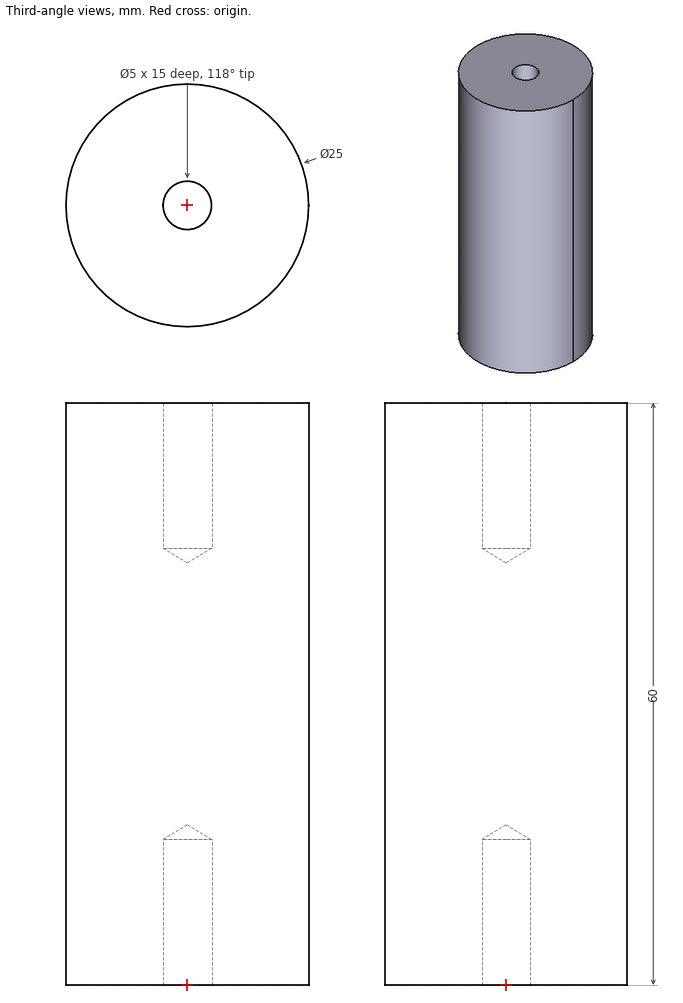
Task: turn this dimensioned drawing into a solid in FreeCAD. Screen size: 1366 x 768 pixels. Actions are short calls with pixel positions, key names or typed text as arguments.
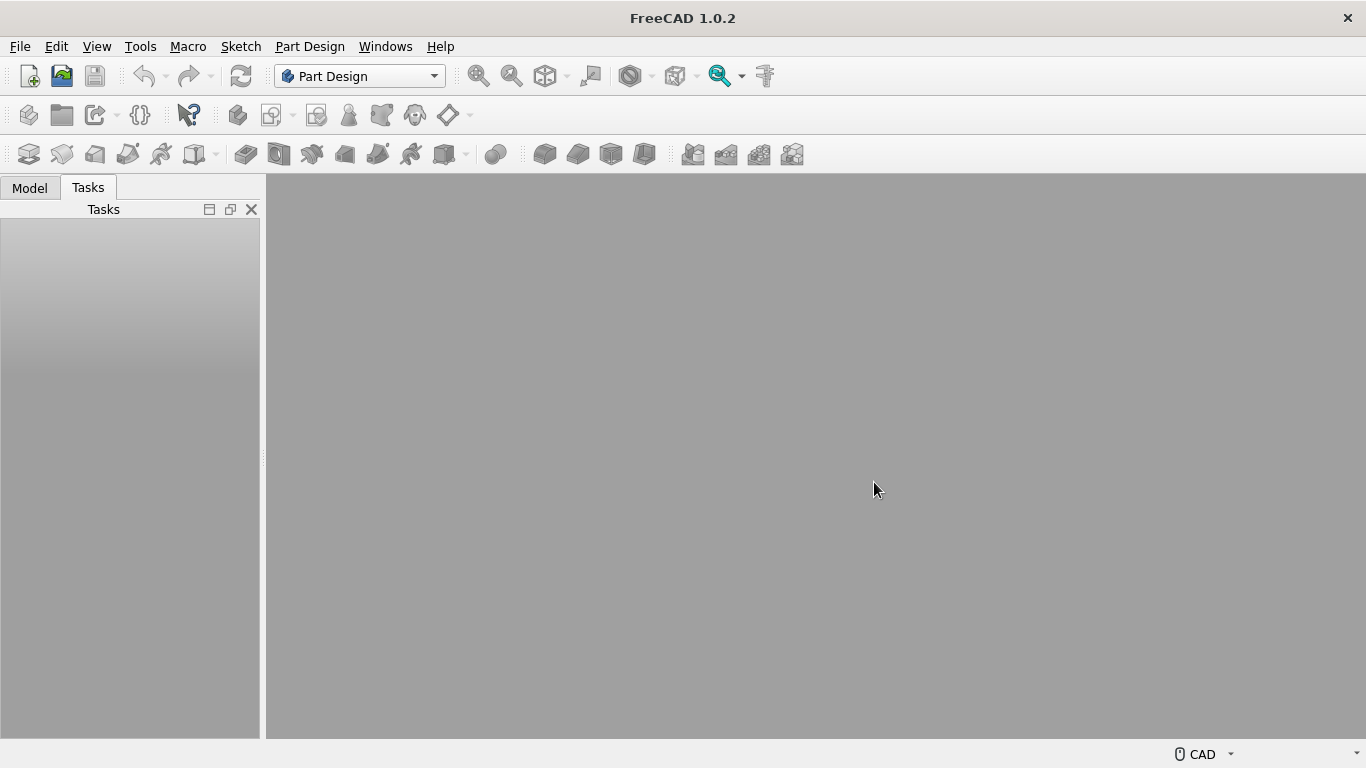
click(29, 76)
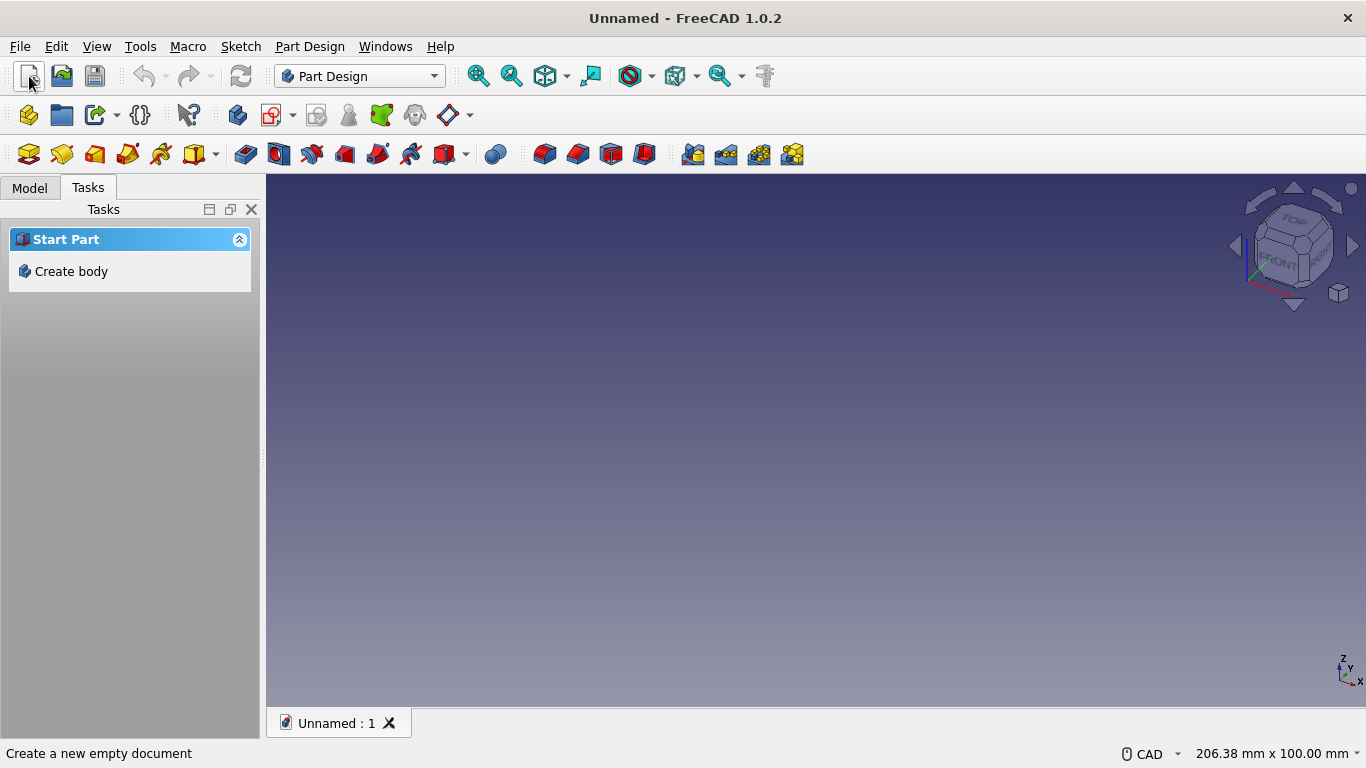
click(270, 116)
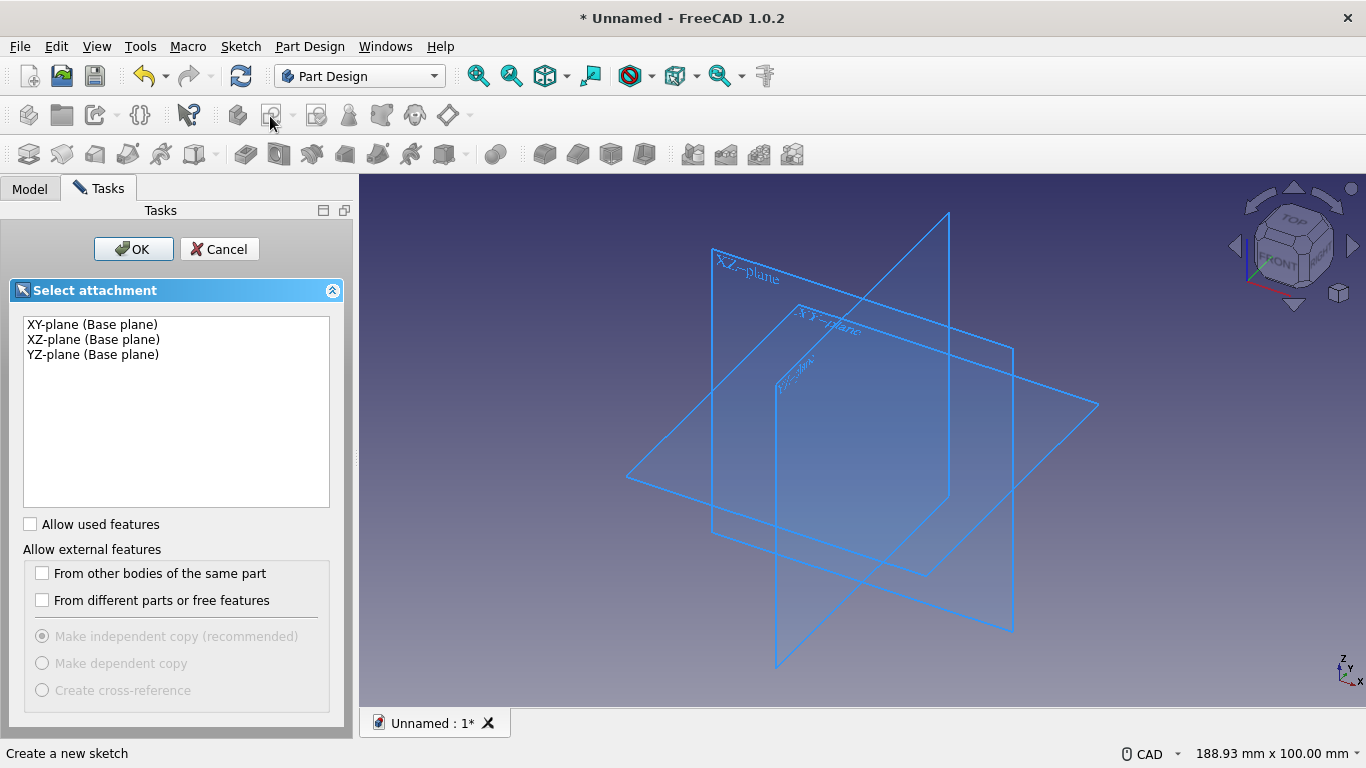
click(84, 324)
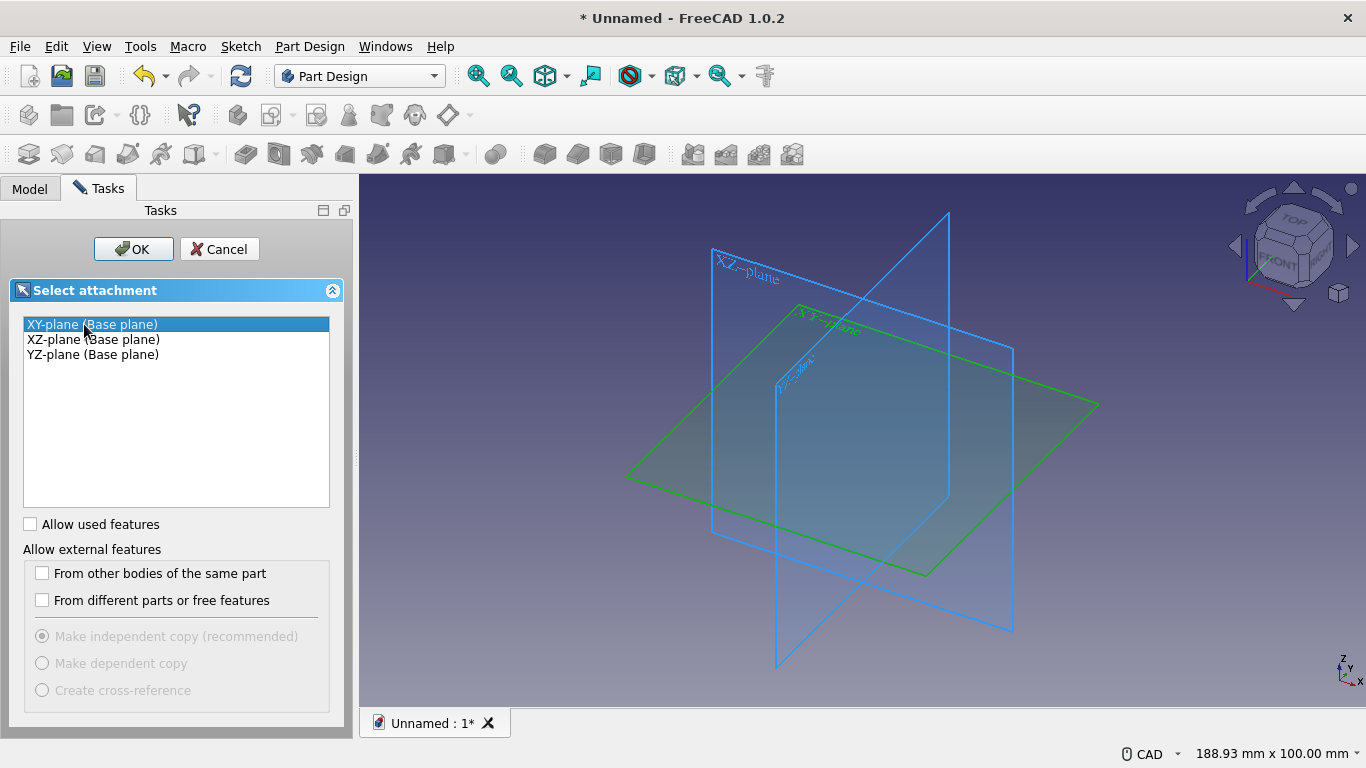
click(134, 249)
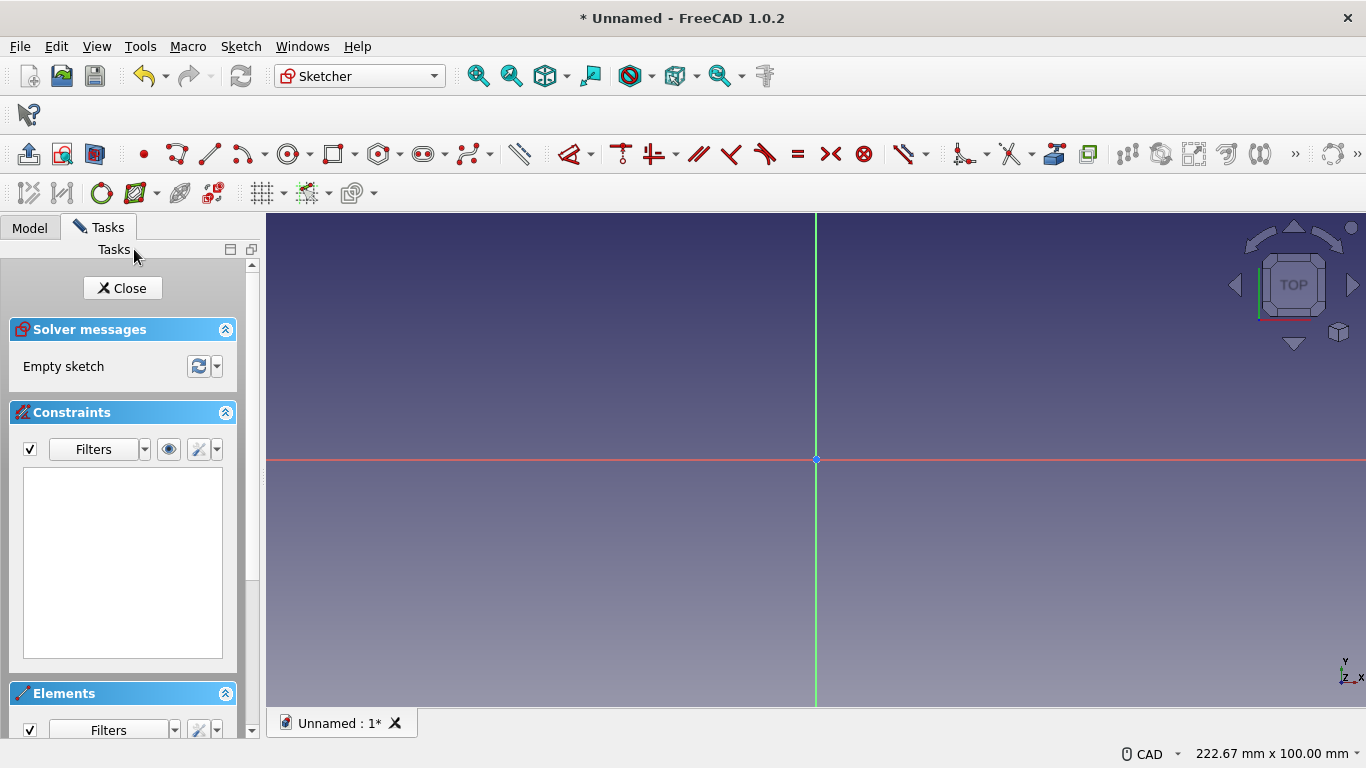
scroll(856, 460, up, 5)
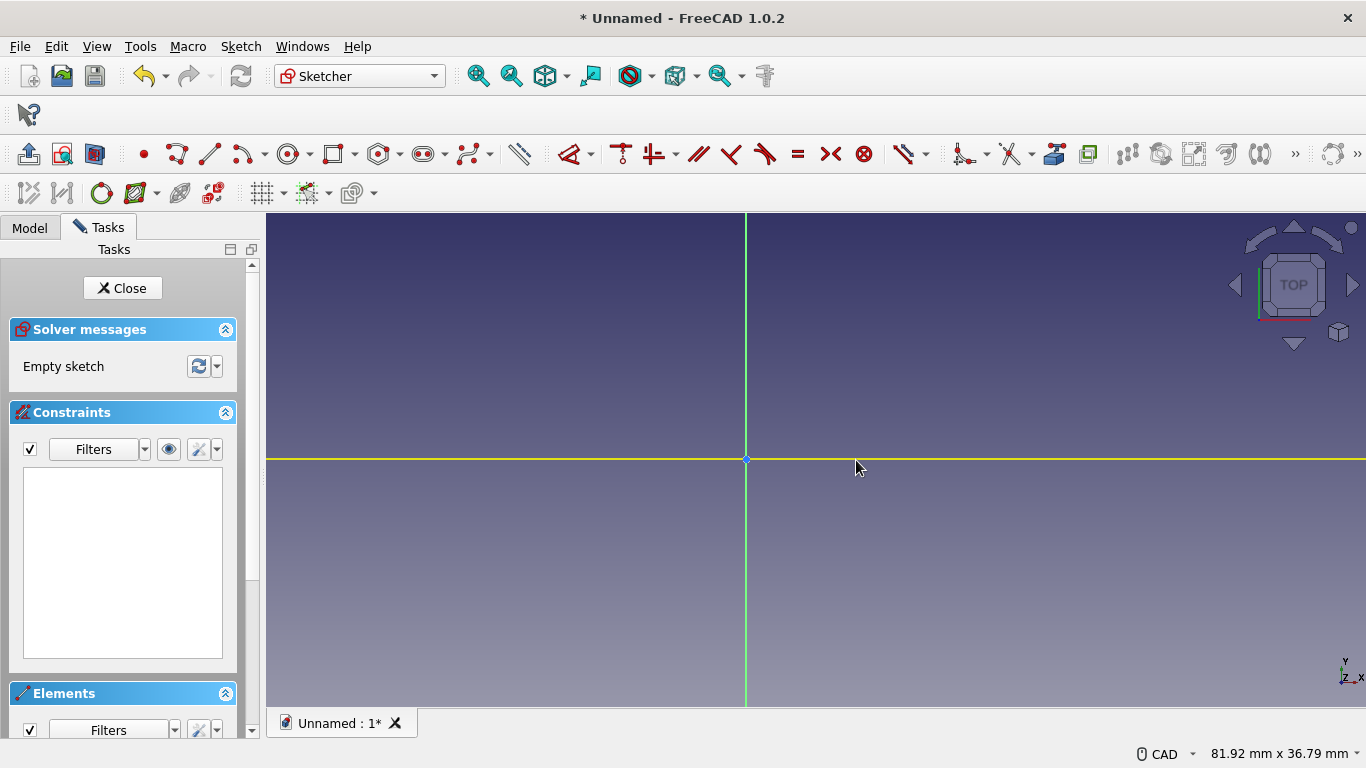
click(288, 154)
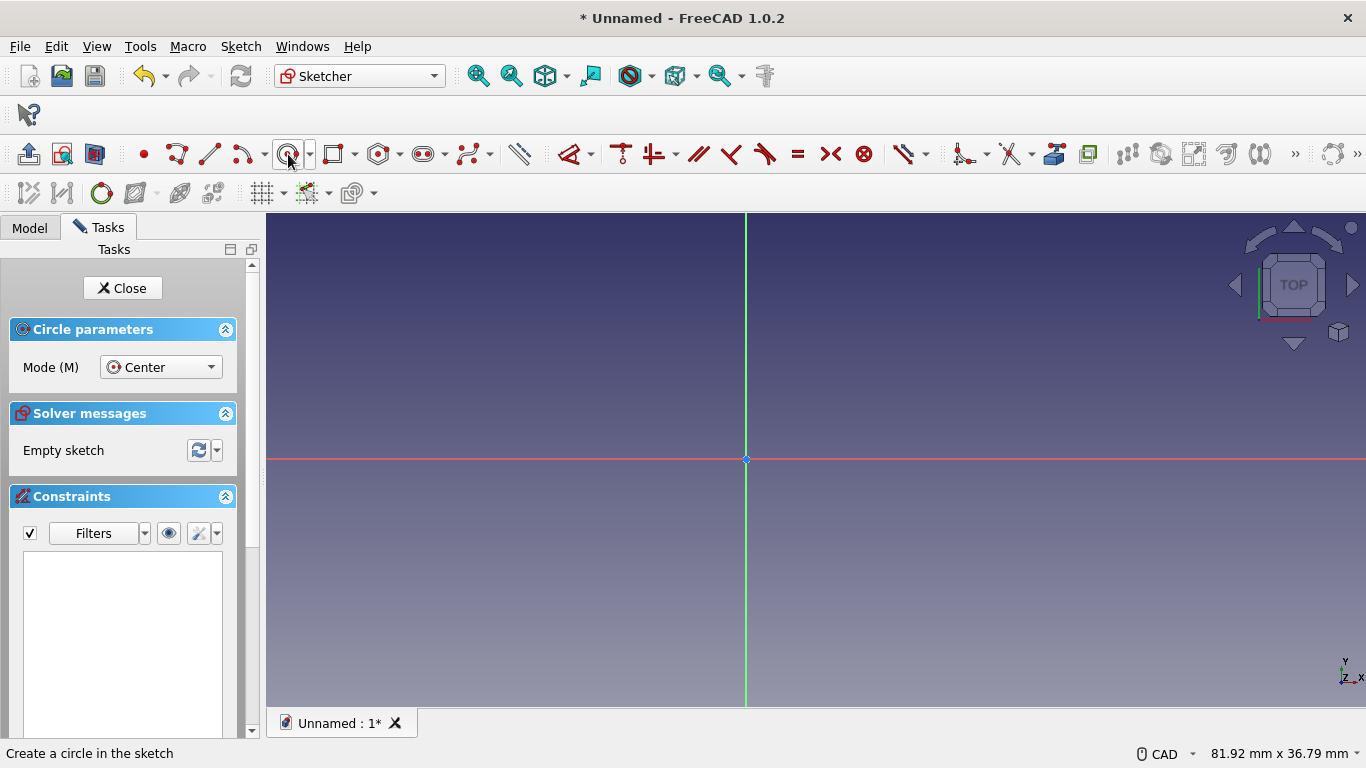
click(746, 459)
click(865, 340)
key(Escape)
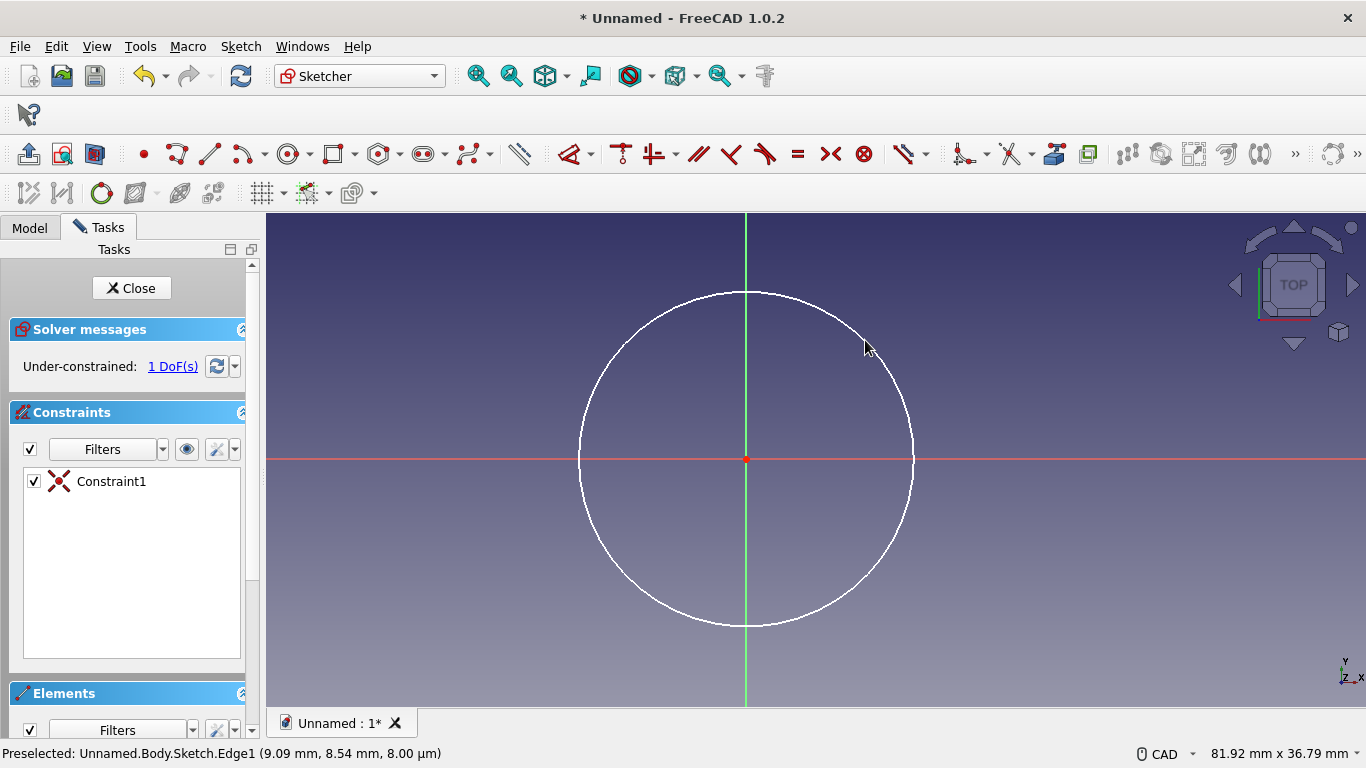
click(568, 154)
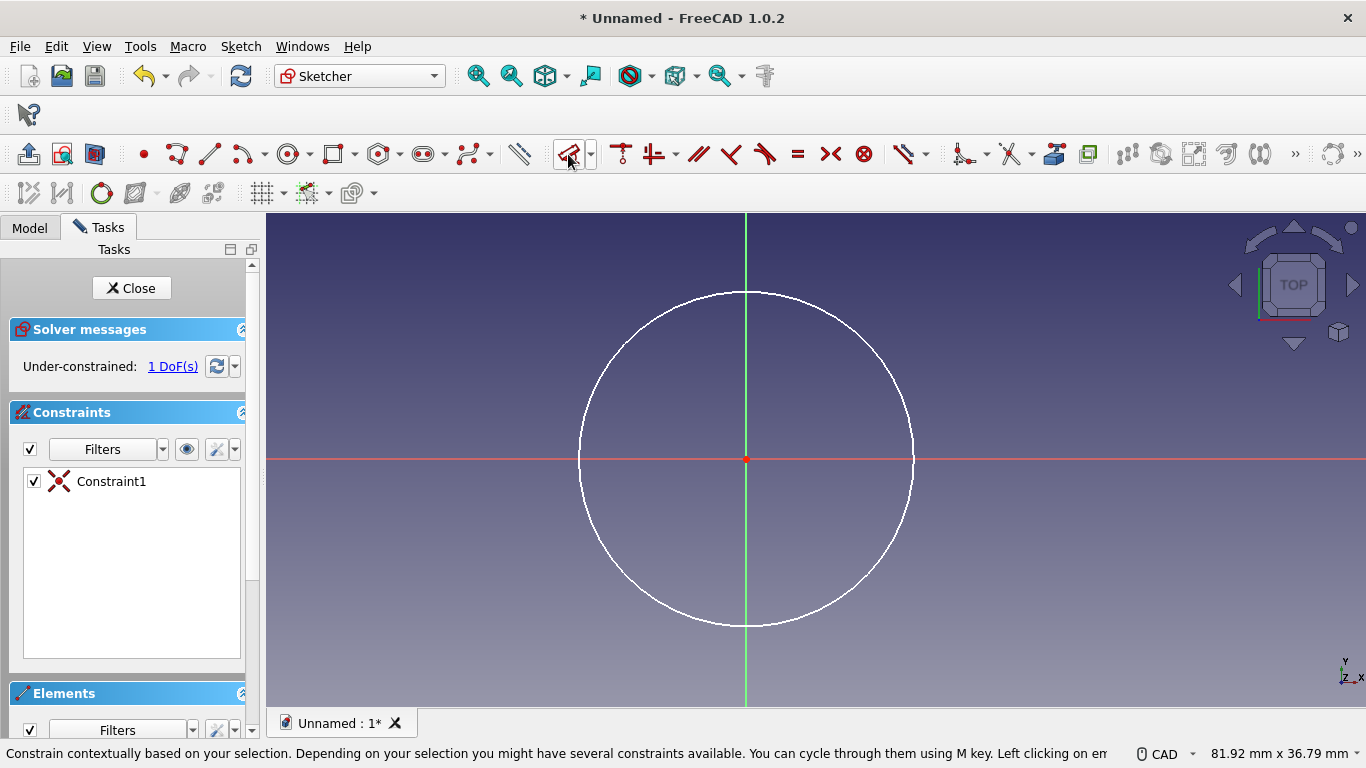
click(864, 340)
click(886, 317)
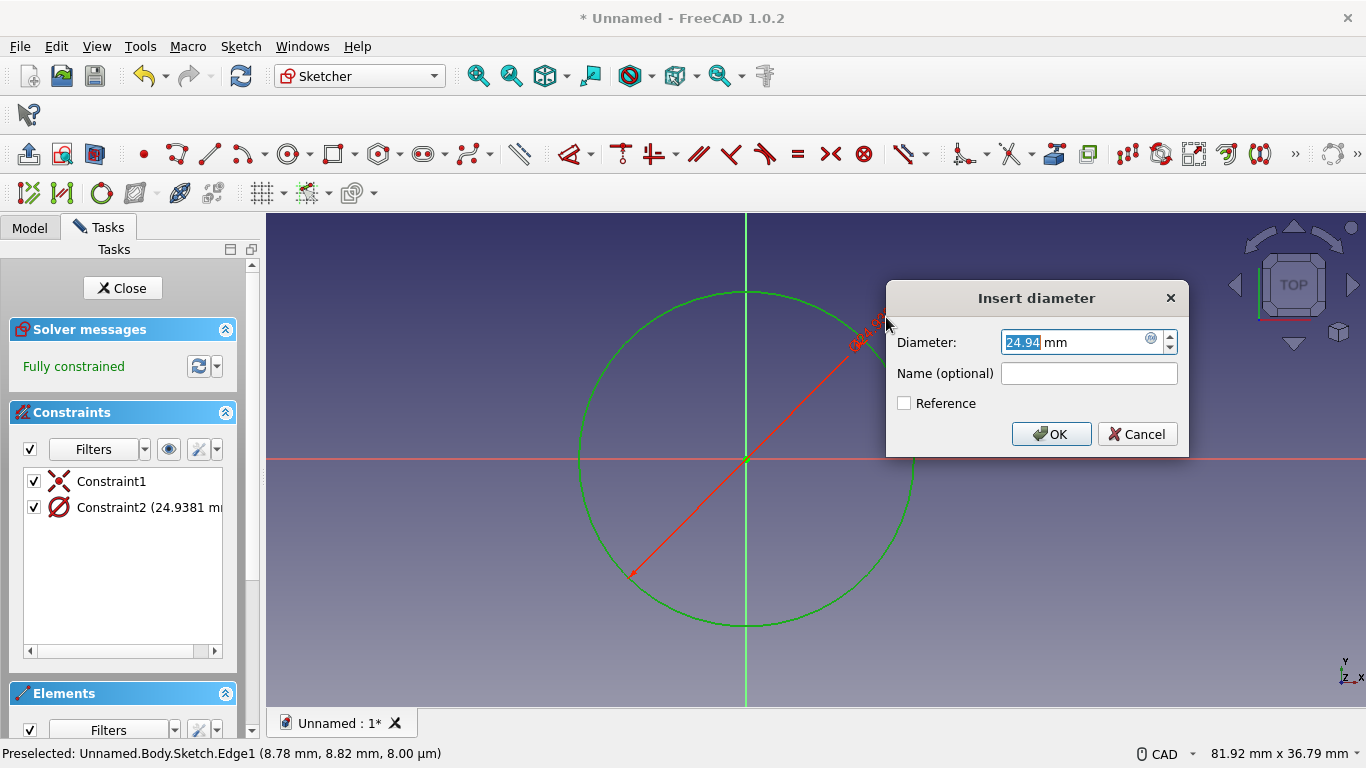
text(25)
key(Return)
key(Escape)